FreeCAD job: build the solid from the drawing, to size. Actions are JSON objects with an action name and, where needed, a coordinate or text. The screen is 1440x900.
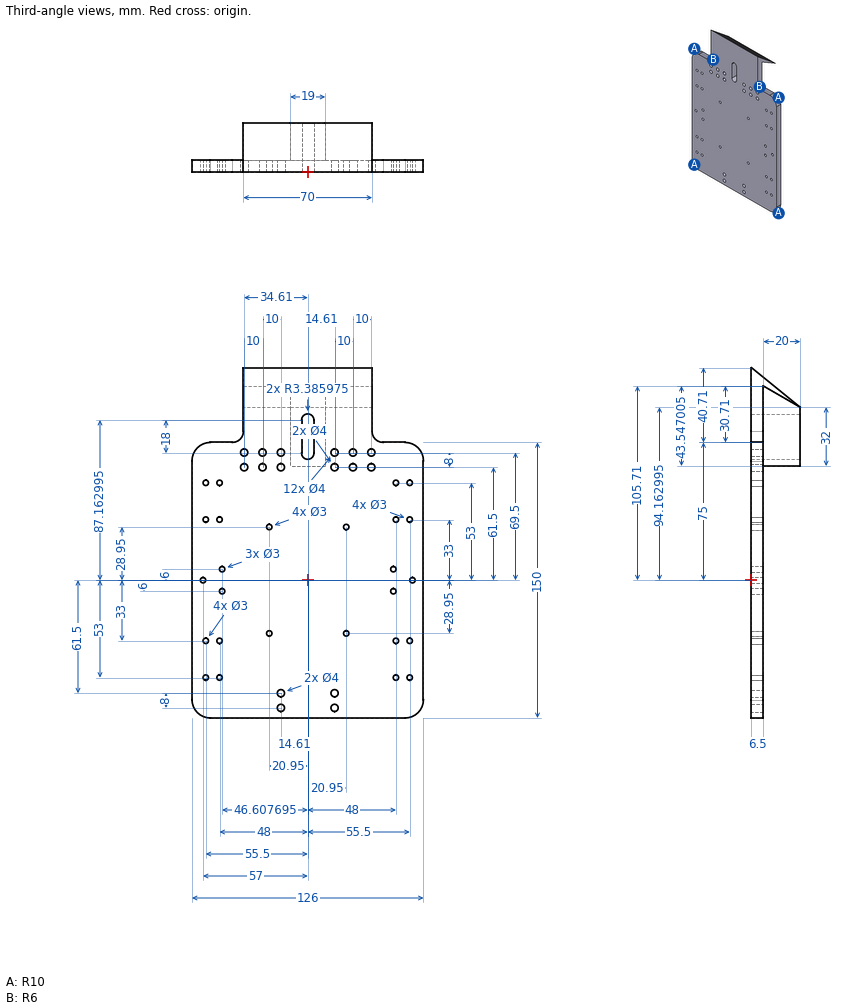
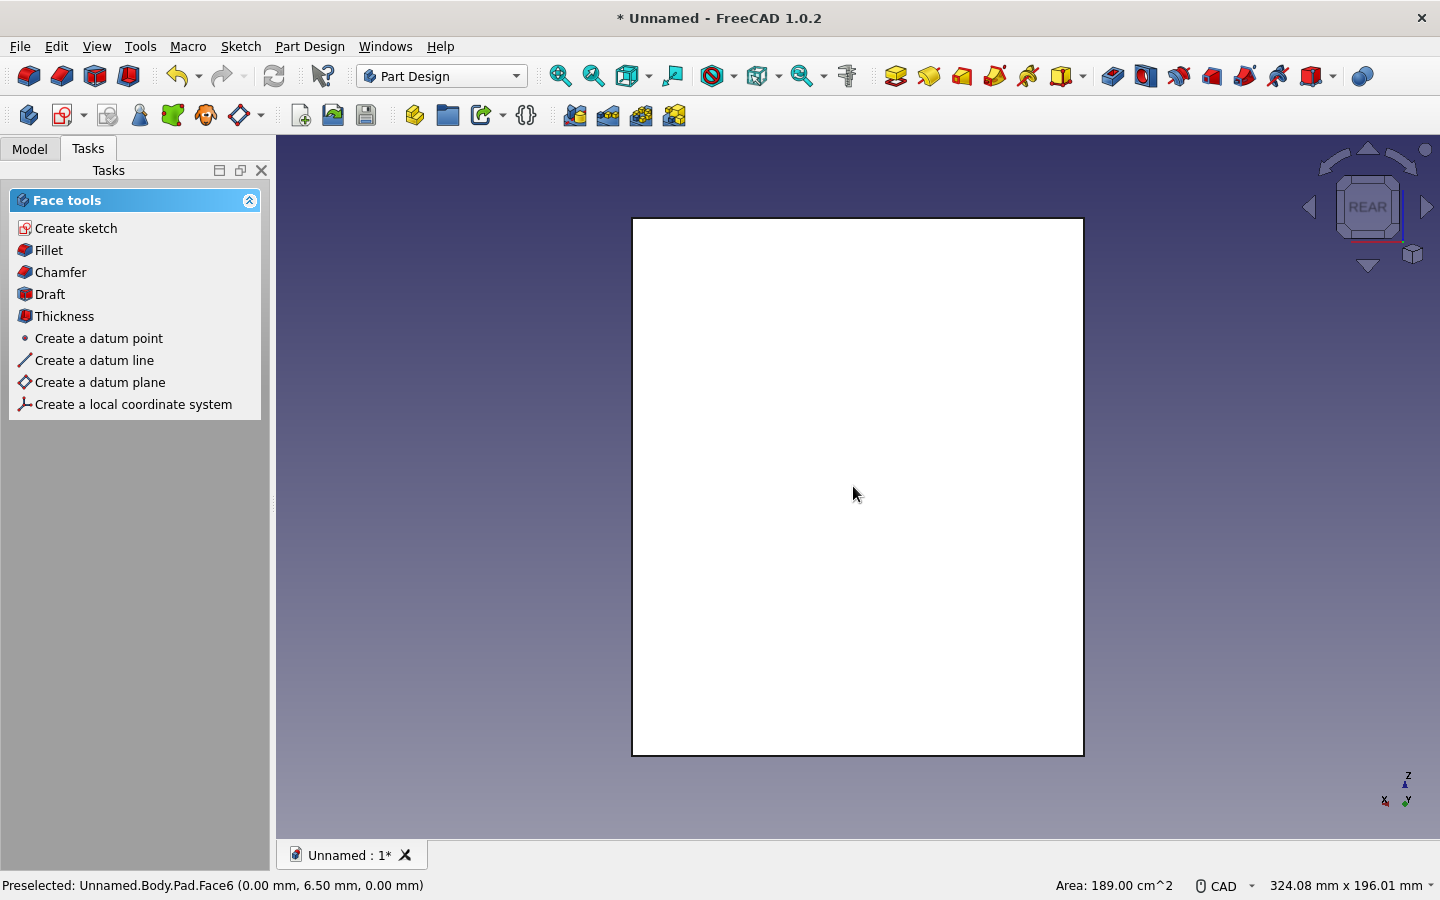
{"action": "left_click", "coordinate": [62, 116]}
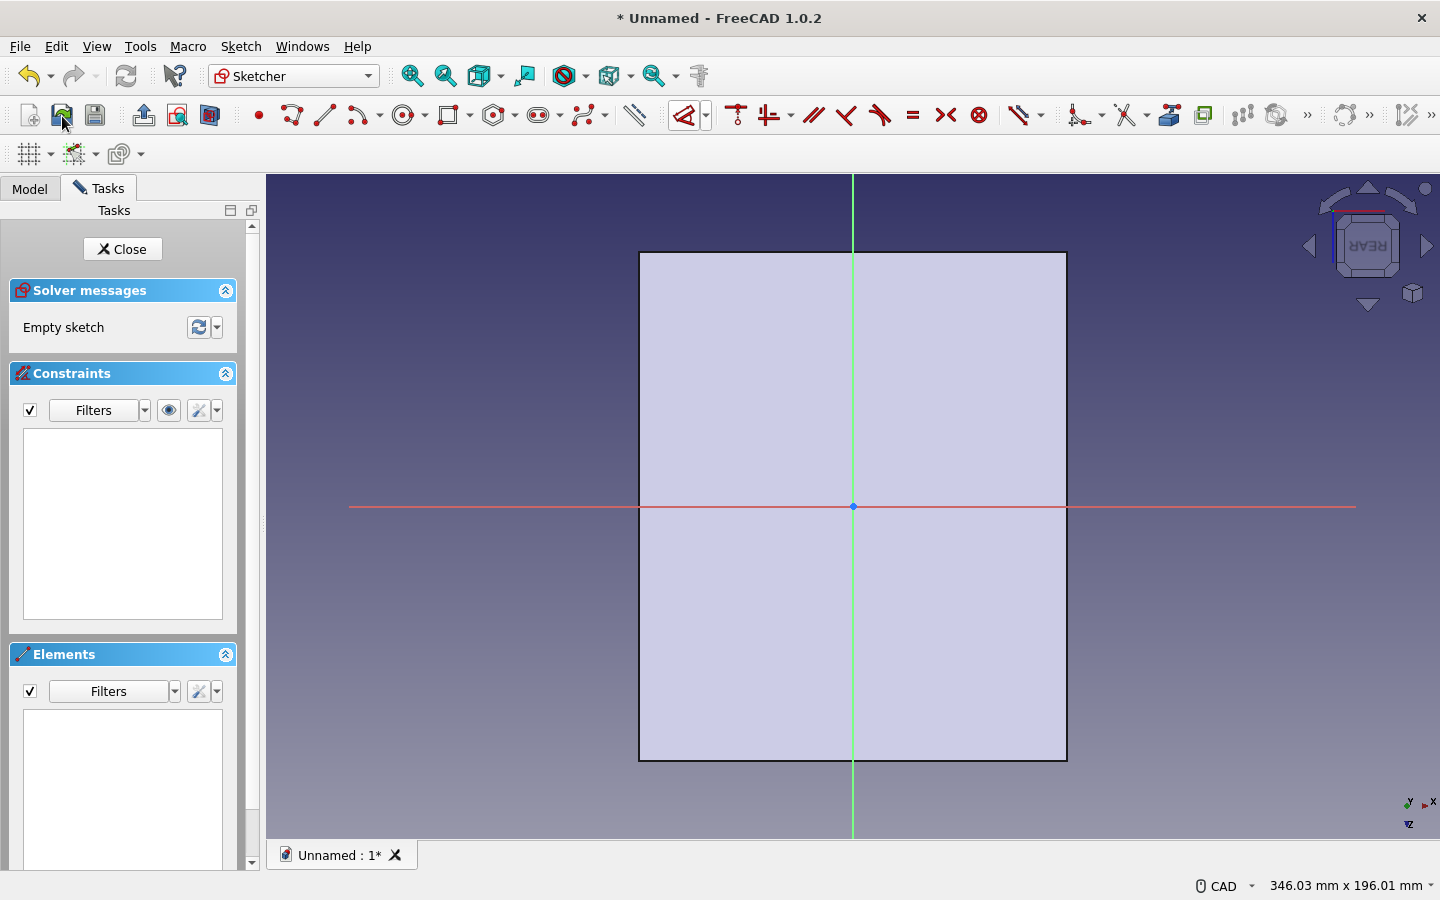
{"action": "scroll", "coordinate": [733, 339], "scroll_direction": "up", "scroll_amount": 4}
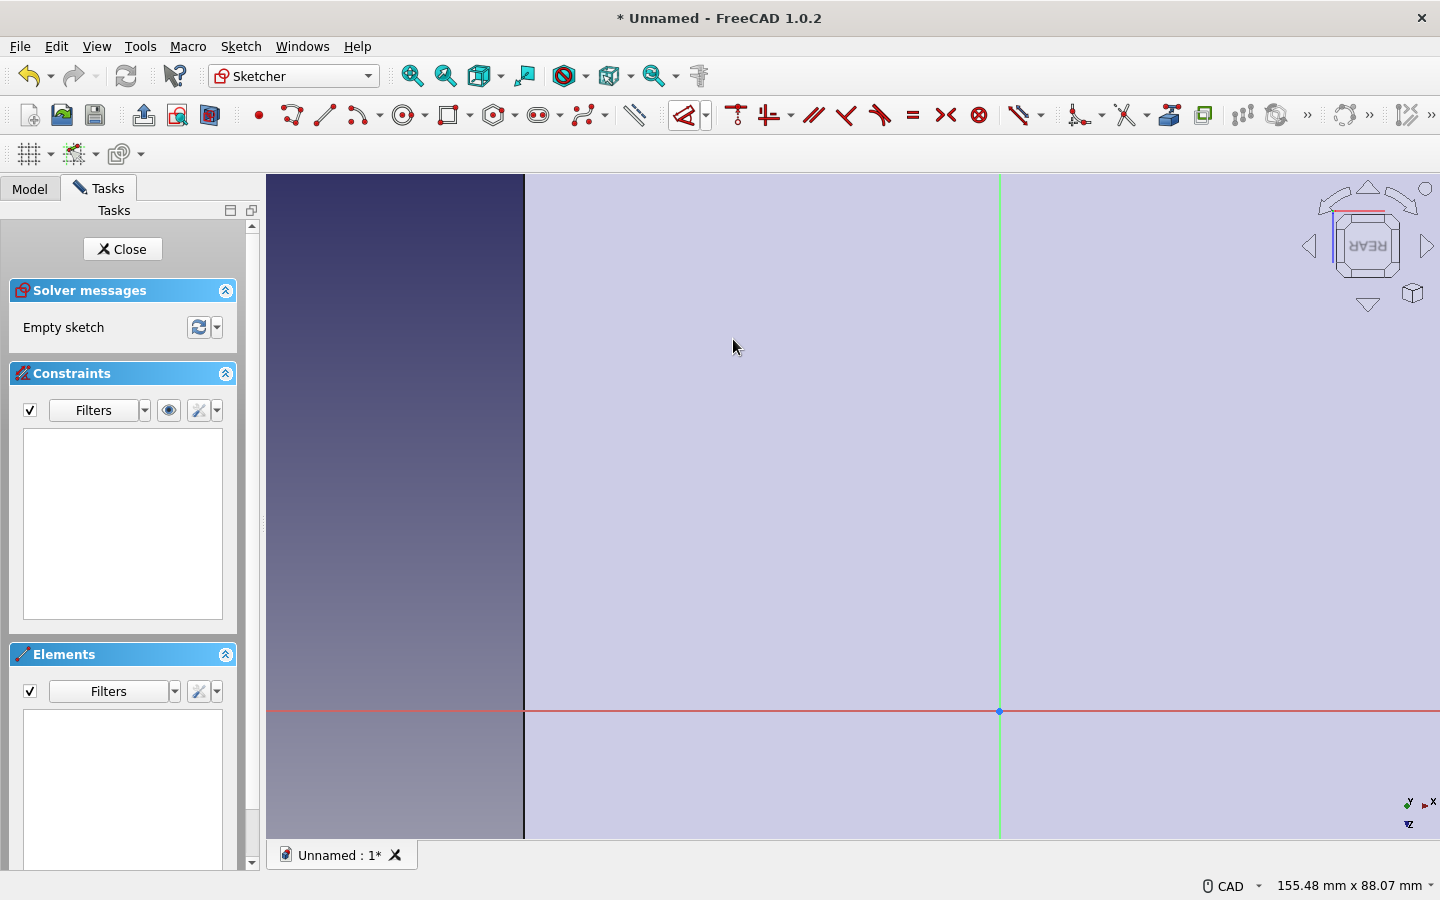
{"action": "left_click", "coordinate": [402, 116]}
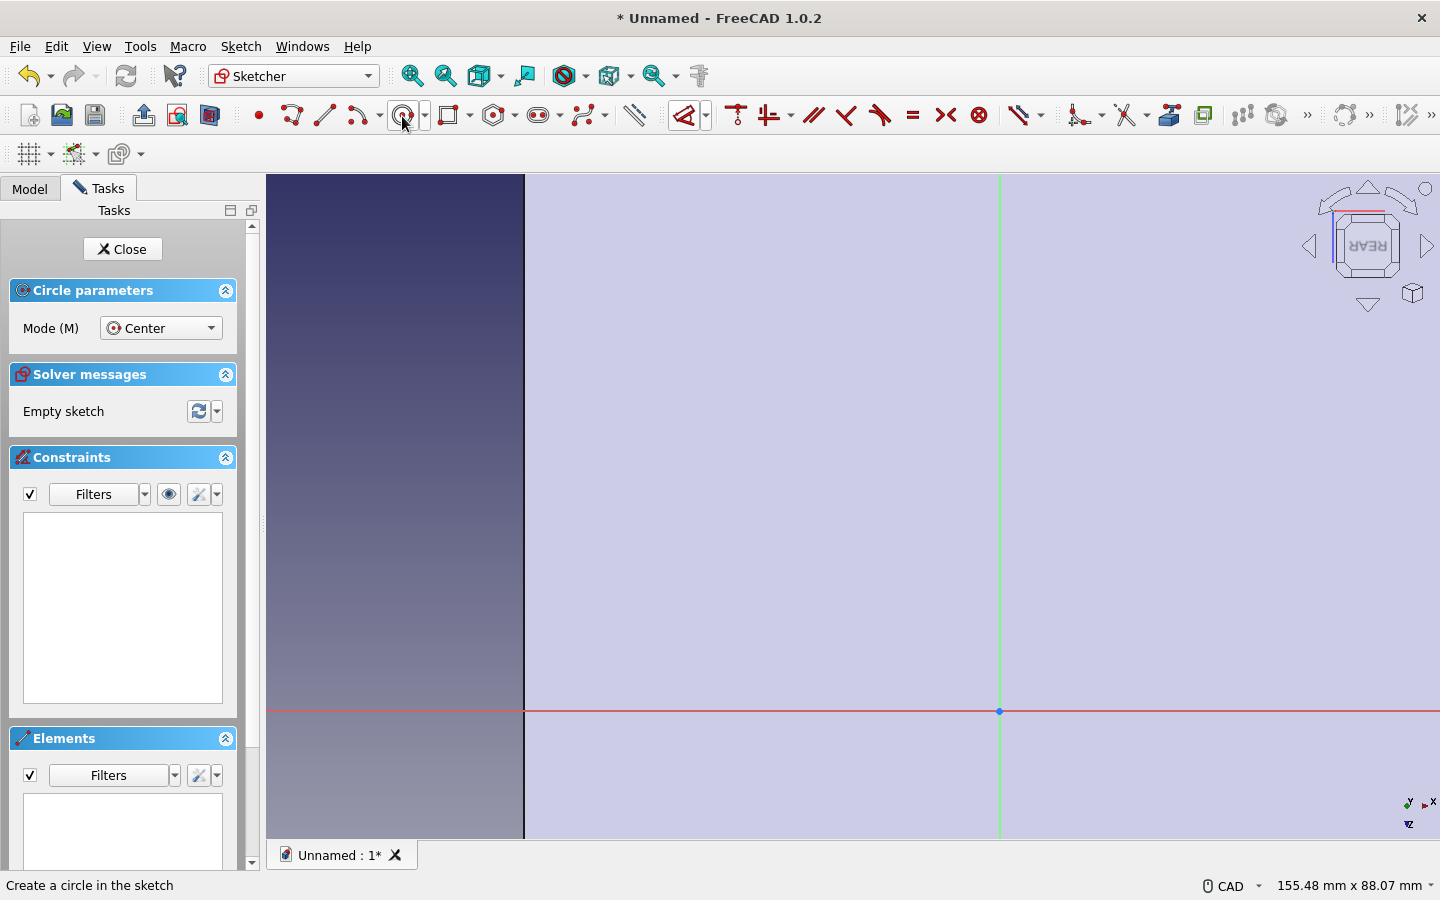
{"action": "scroll", "coordinate": [581, 462], "scroll_direction": "up", "scroll_amount": 4}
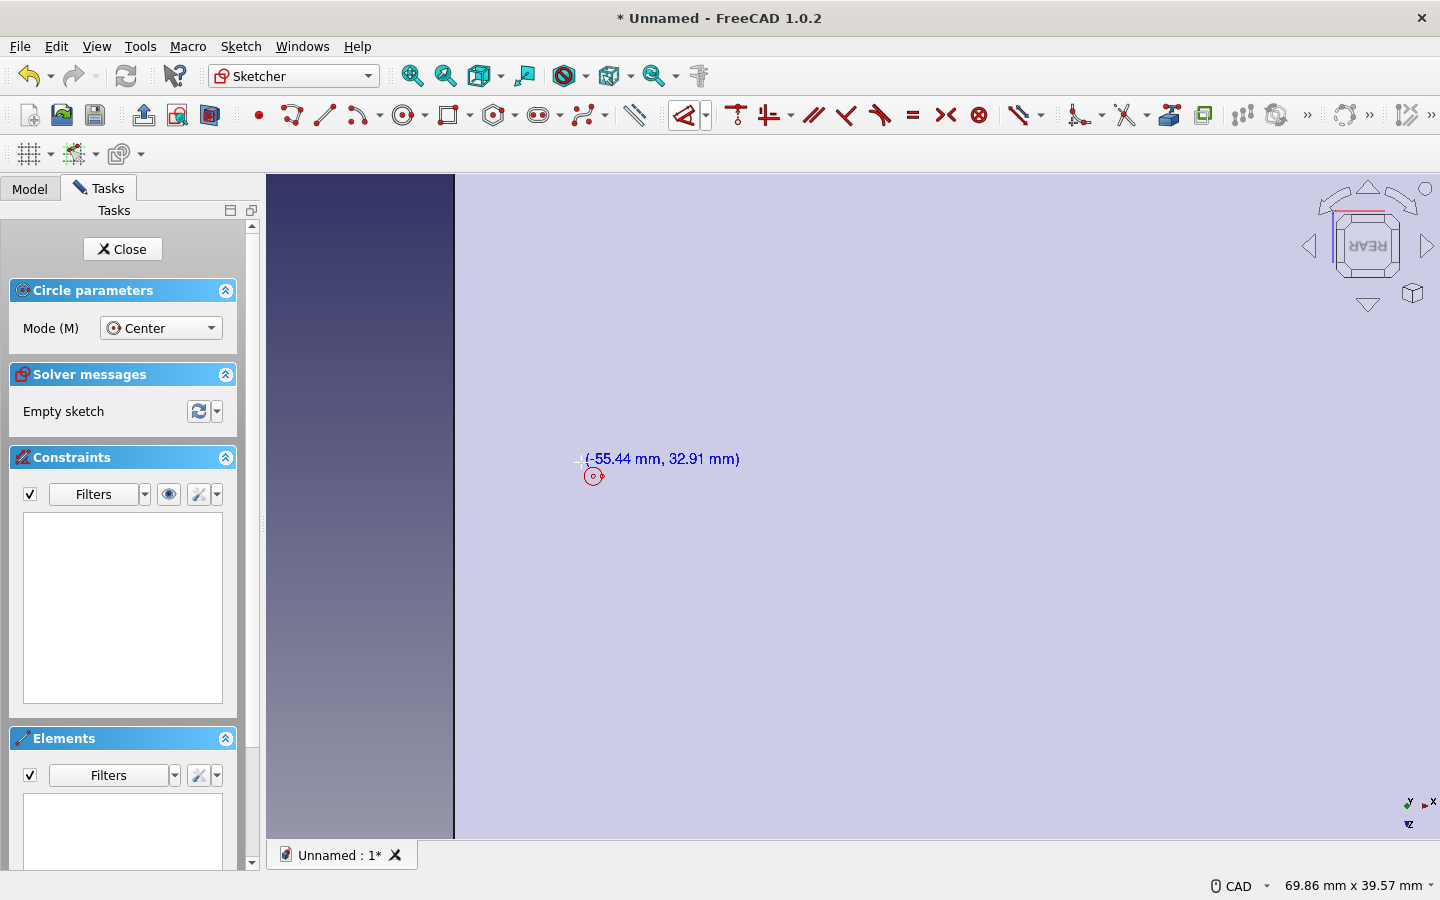
{"action": "left_click", "coordinate": [580, 462]}
{"action": "mouse_move", "coordinate": [597, 444]}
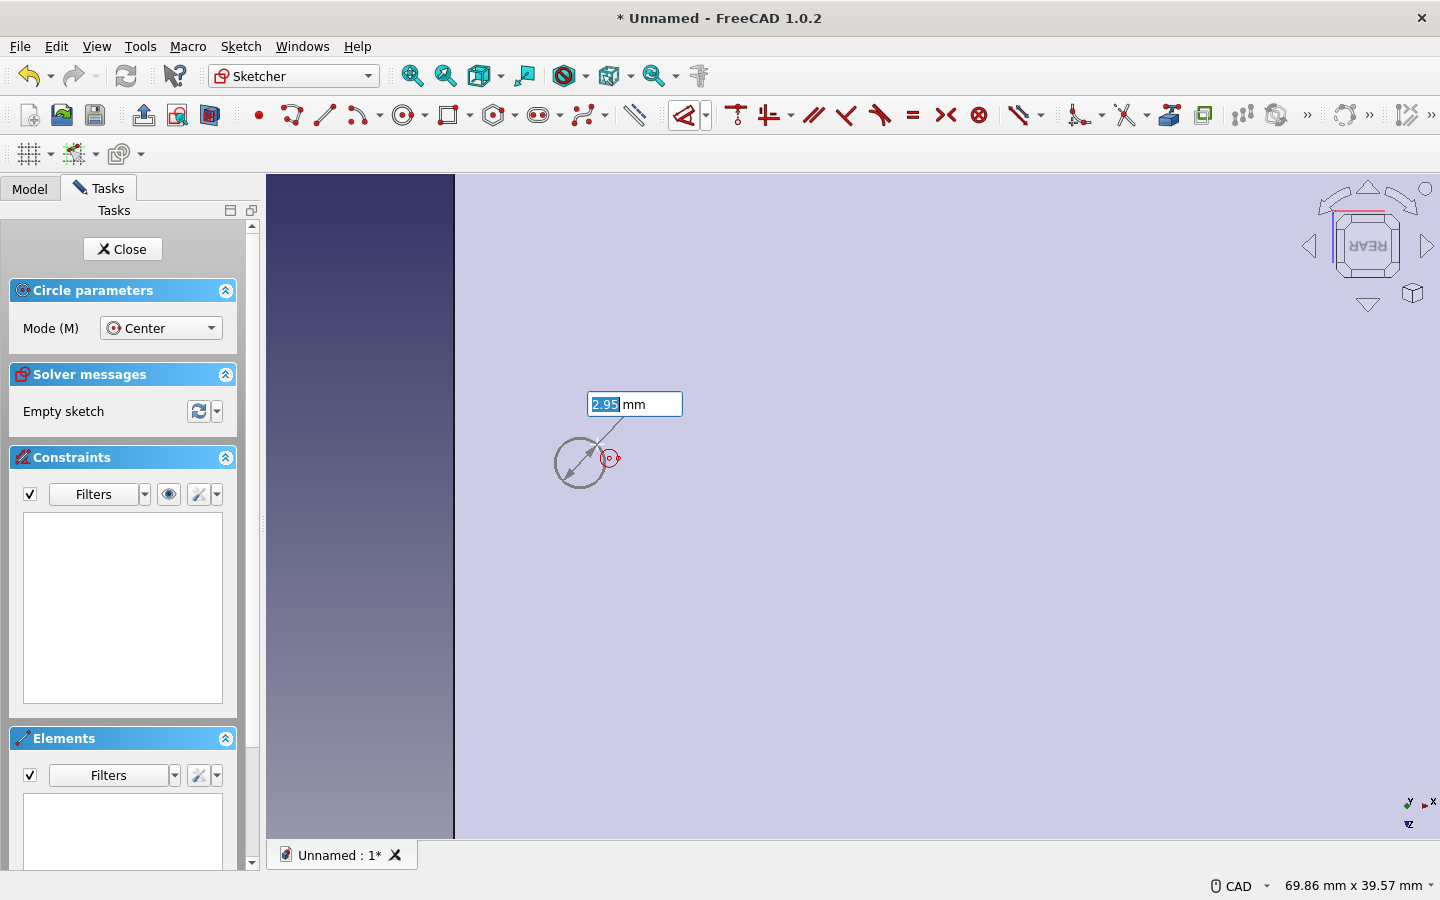
{"action": "type", "text": "3"}
{"action": "key", "text": "Return"}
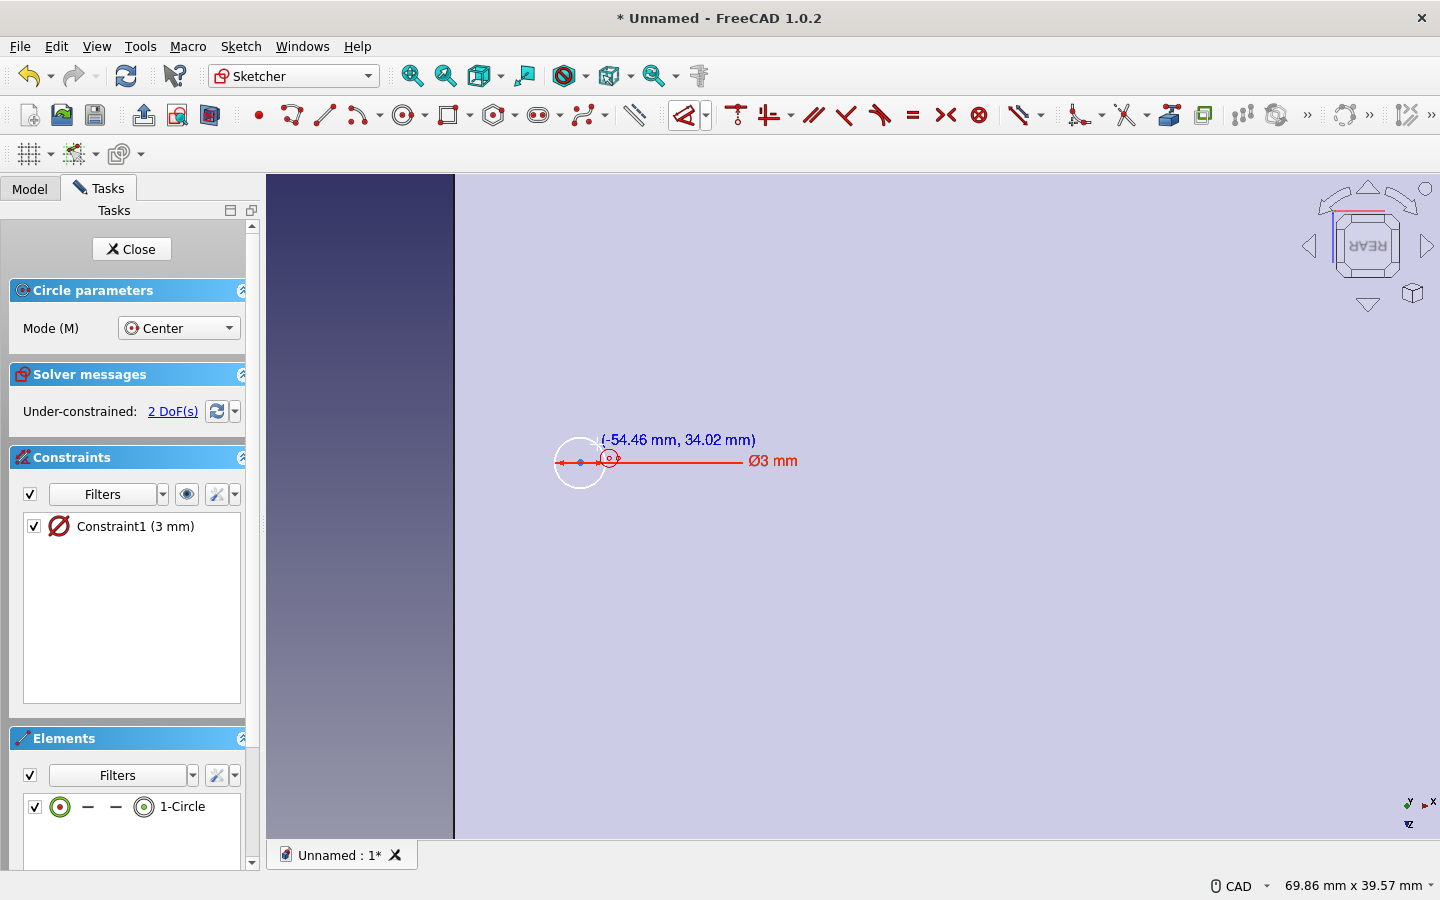
{"action": "left_click", "coordinate": [706, 462]}
{"action": "mouse_move", "coordinate": [723, 444]}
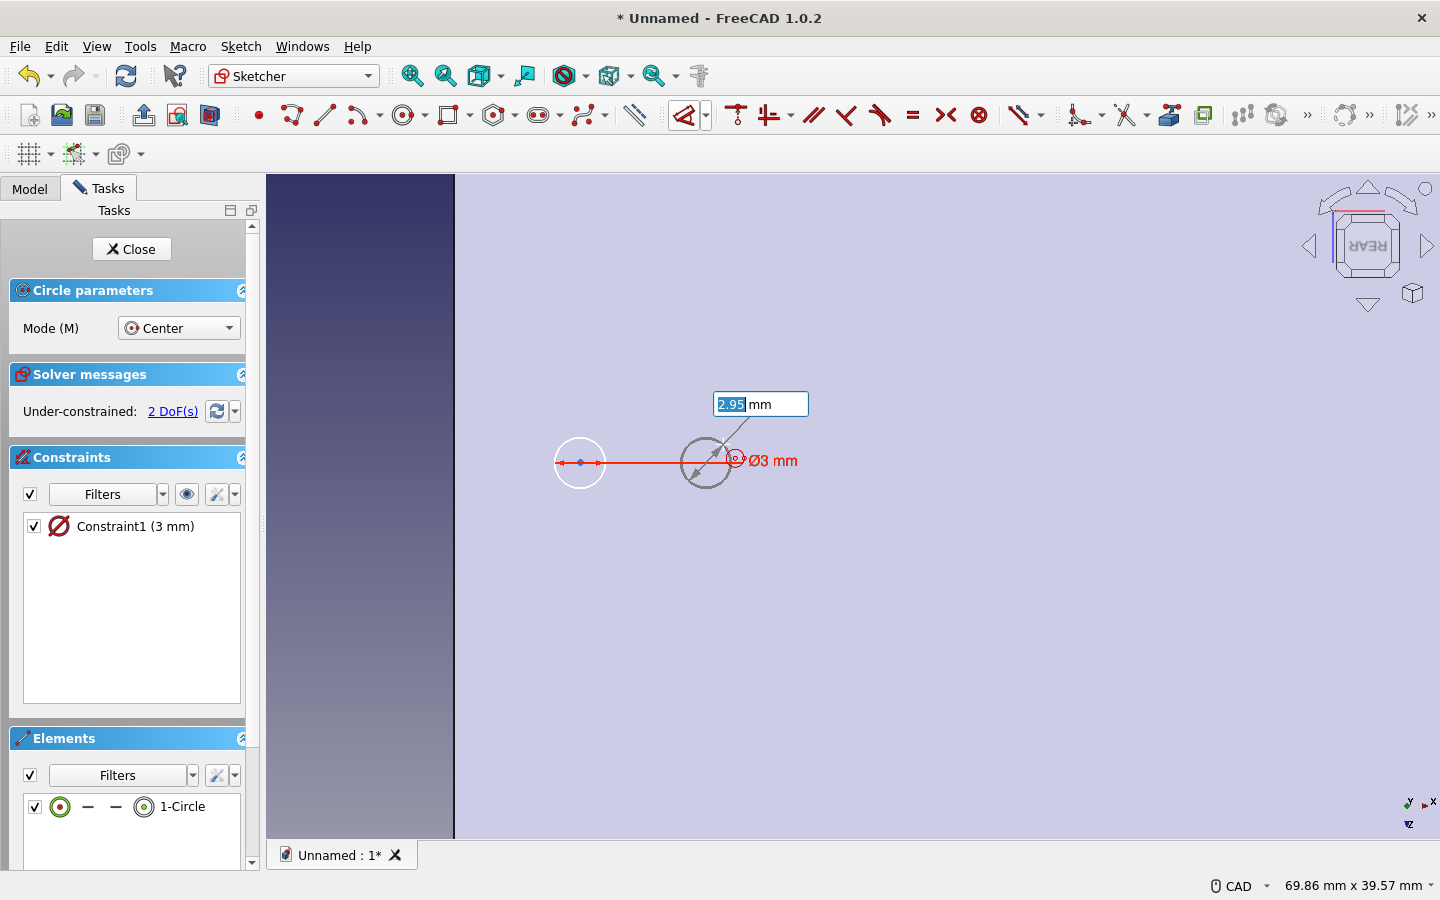
{"action": "type", "text": "3"}
{"action": "key", "text": "Return"}